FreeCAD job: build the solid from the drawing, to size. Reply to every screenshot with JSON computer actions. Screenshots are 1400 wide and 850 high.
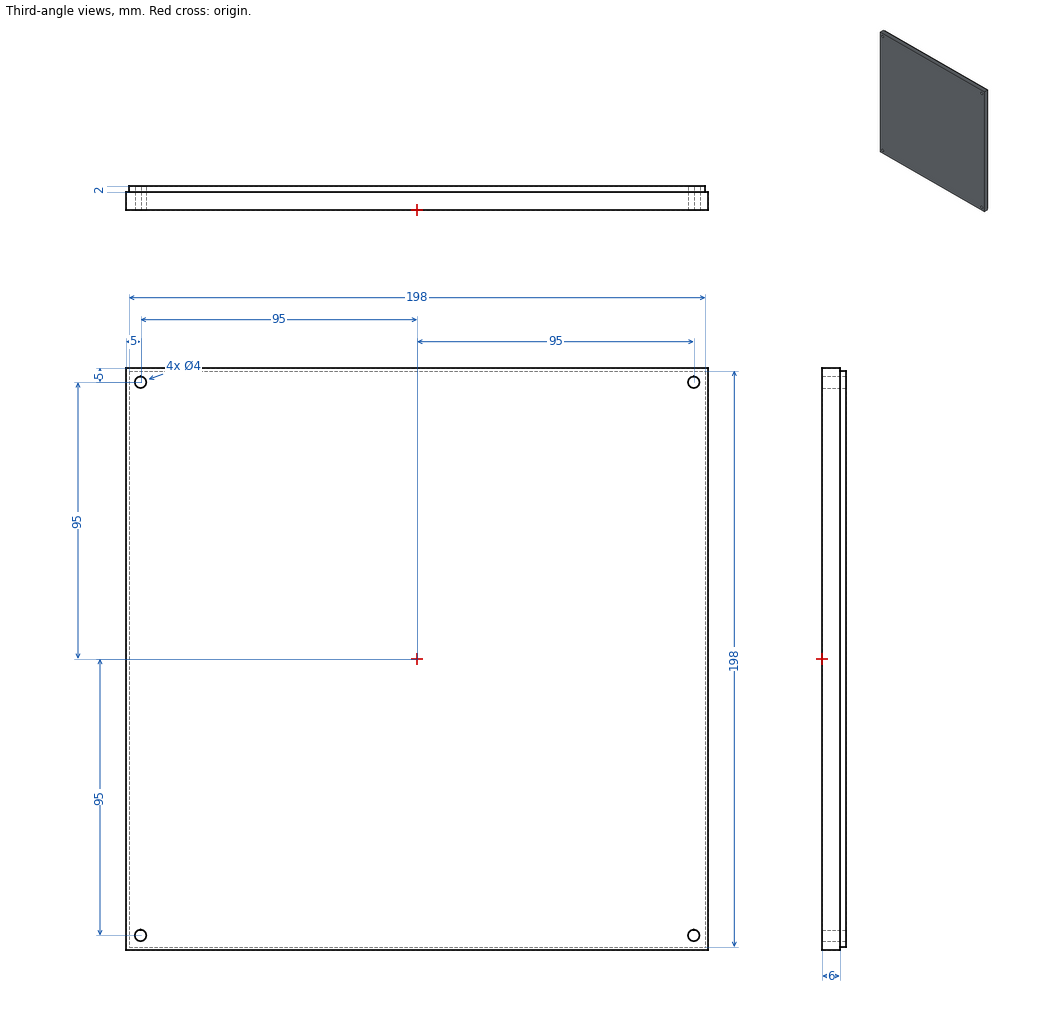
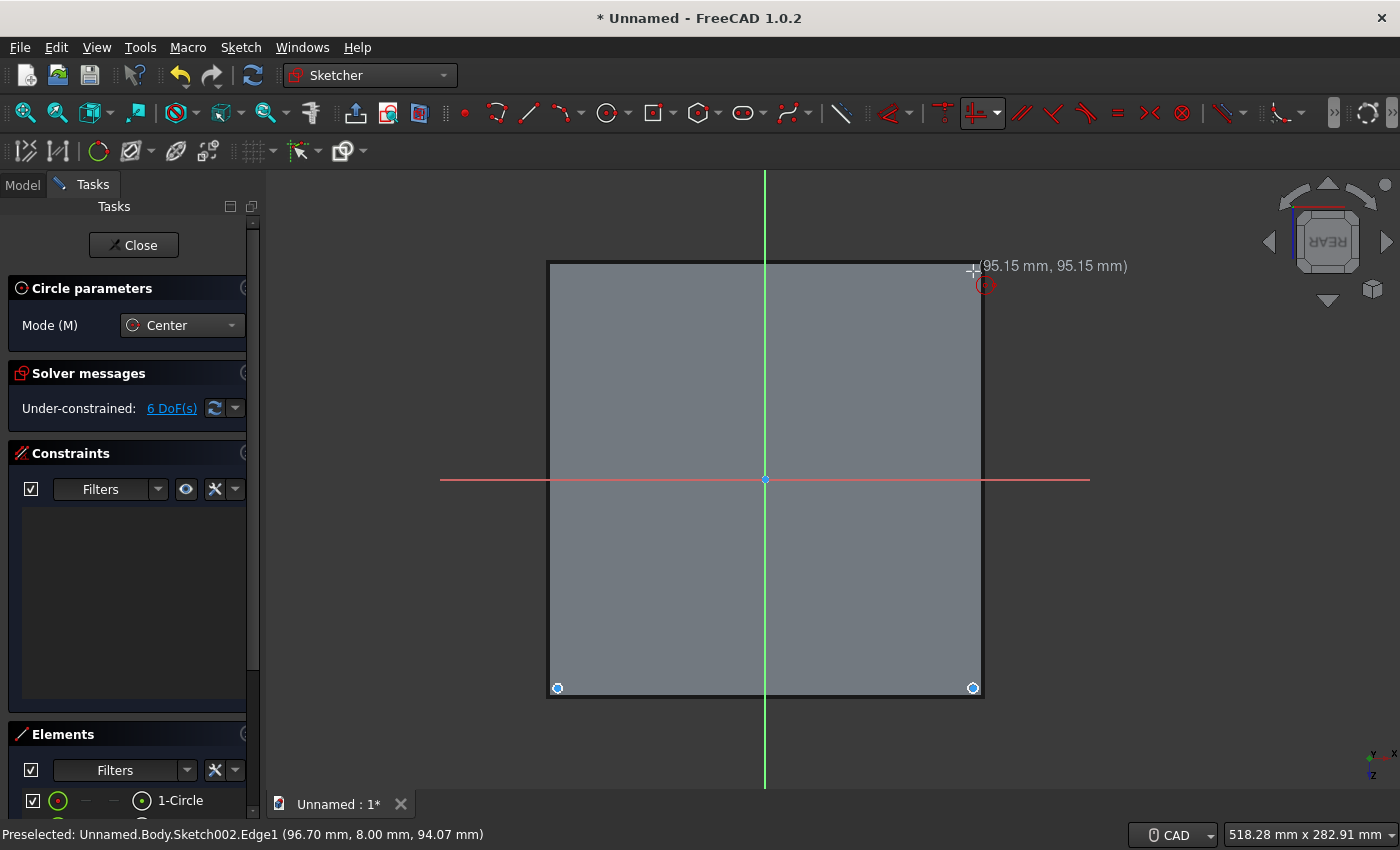
{"action": "left_click", "coordinate": [973, 272]}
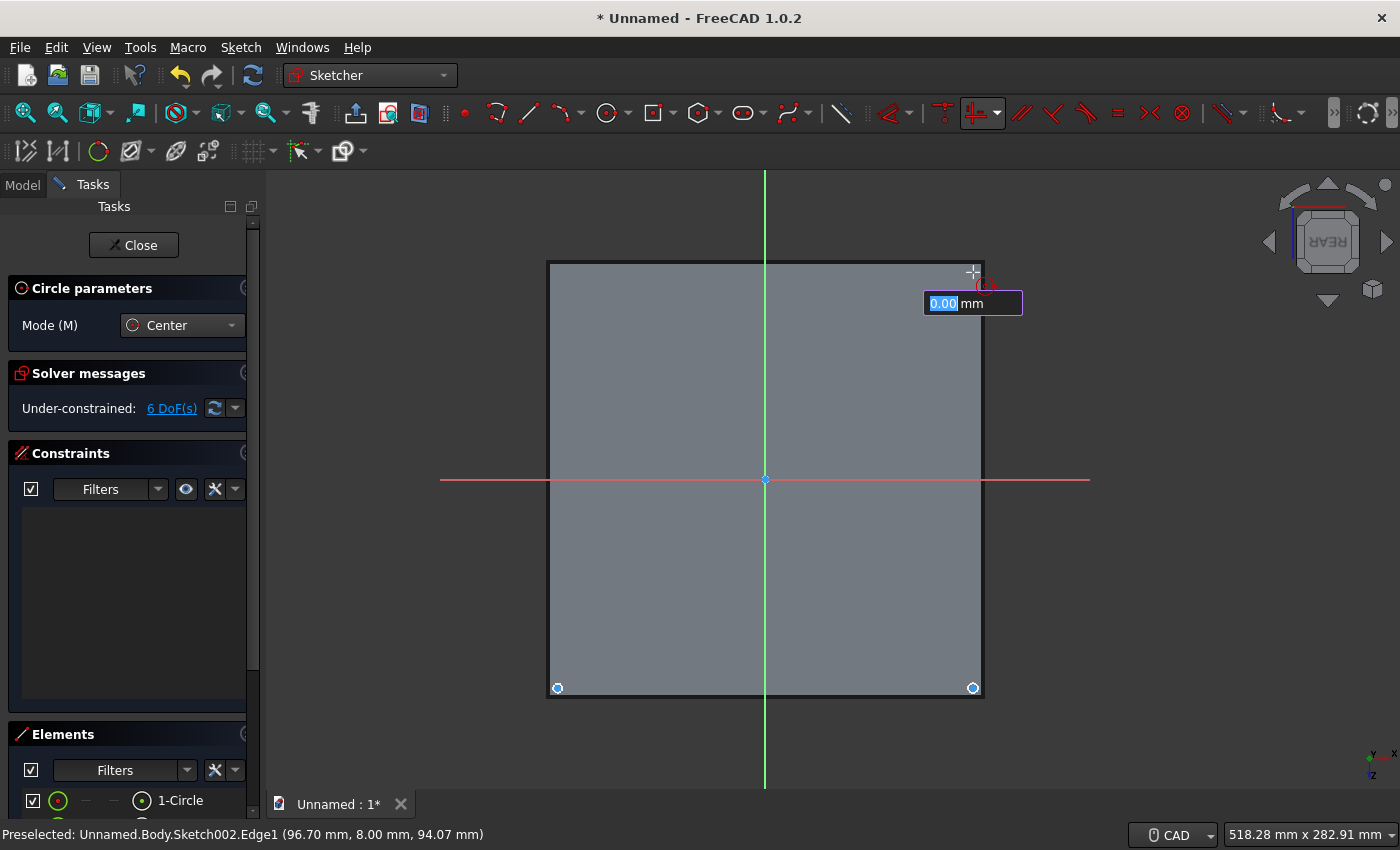
{"action": "scroll", "coordinate": [976, 269], "scroll_direction": "up", "scroll_amount": 7}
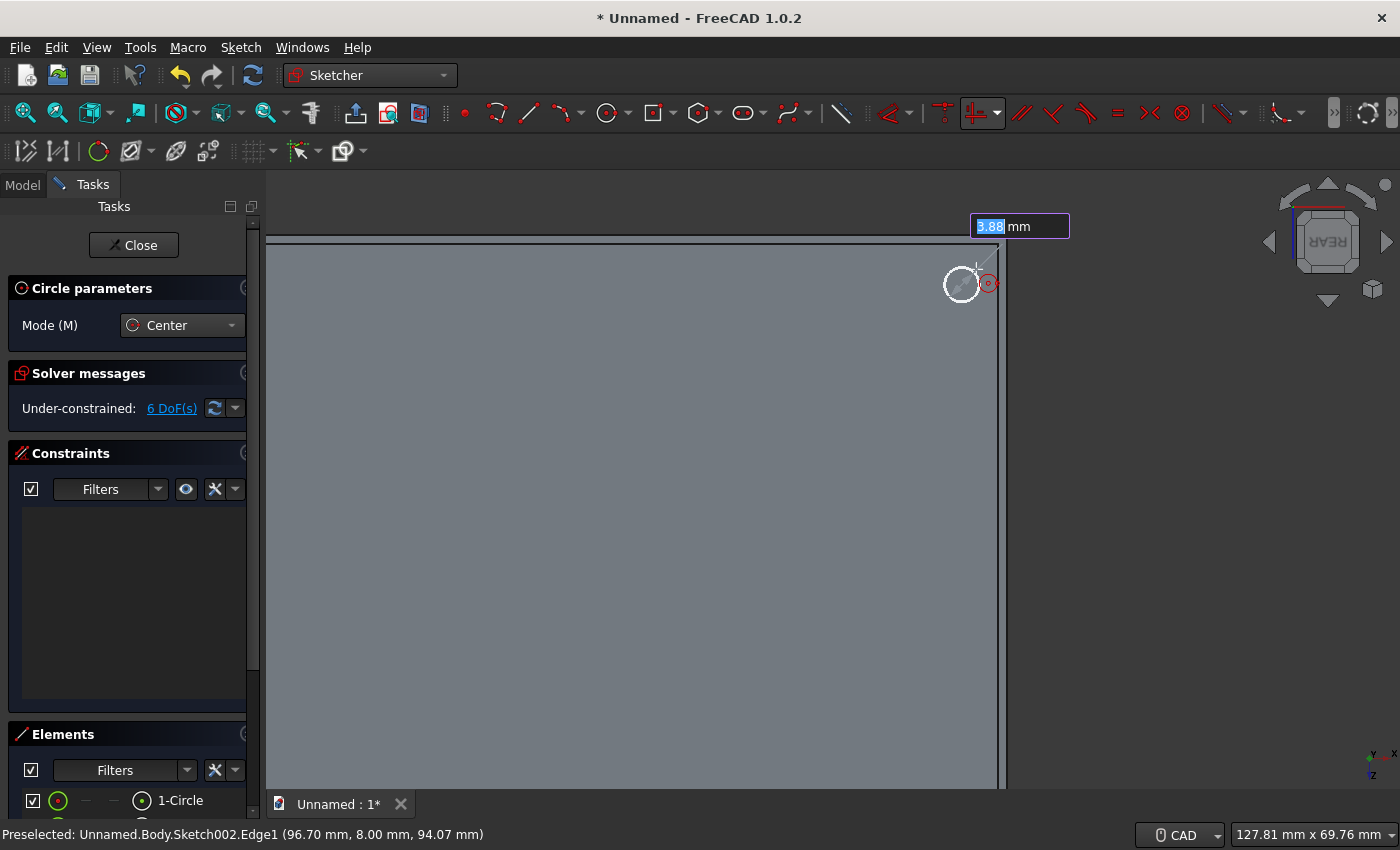
{"action": "left_click", "coordinate": [975, 267]}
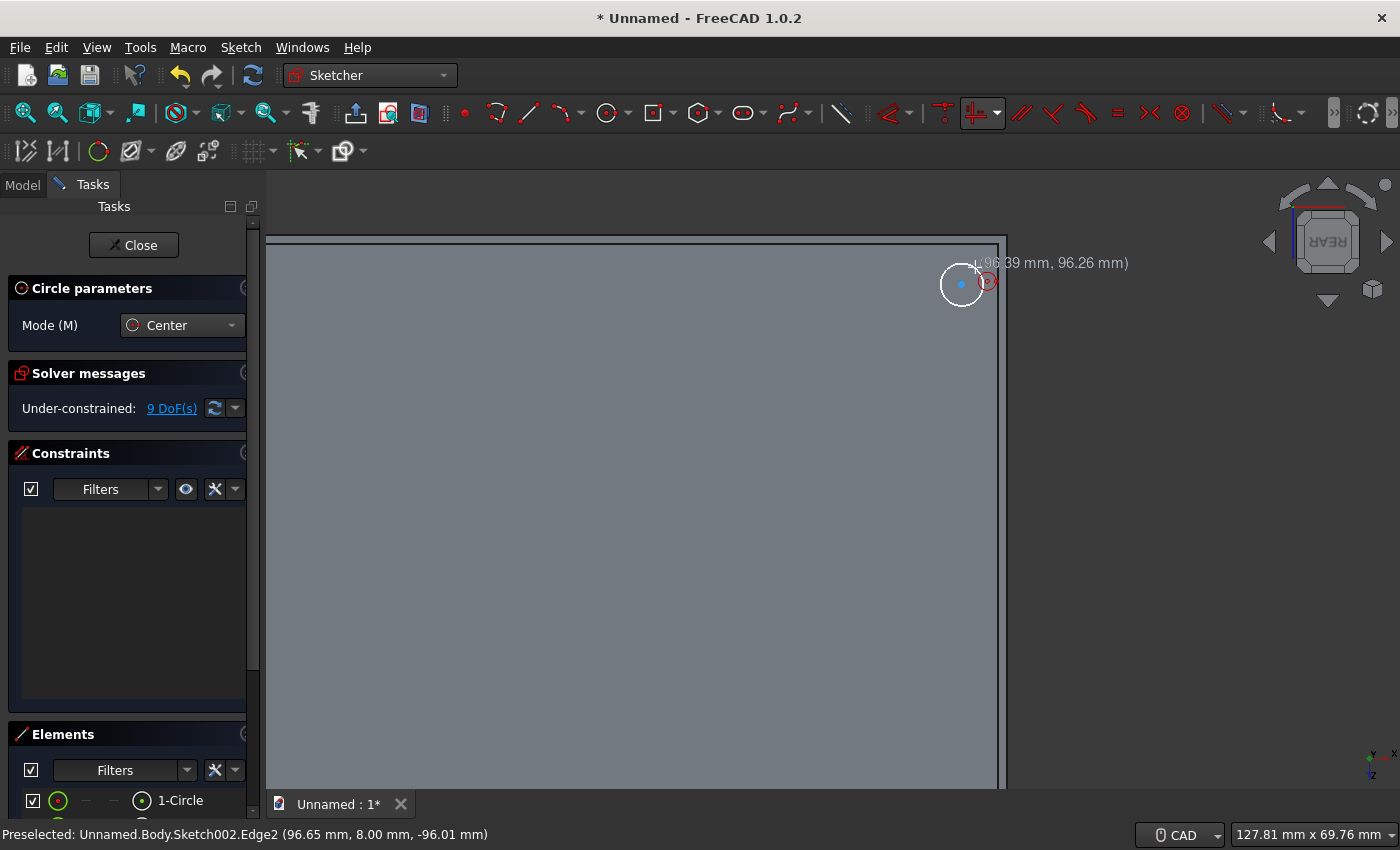
{"action": "scroll", "coordinate": [976, 269], "scroll_direction": "down", "scroll_amount": 7}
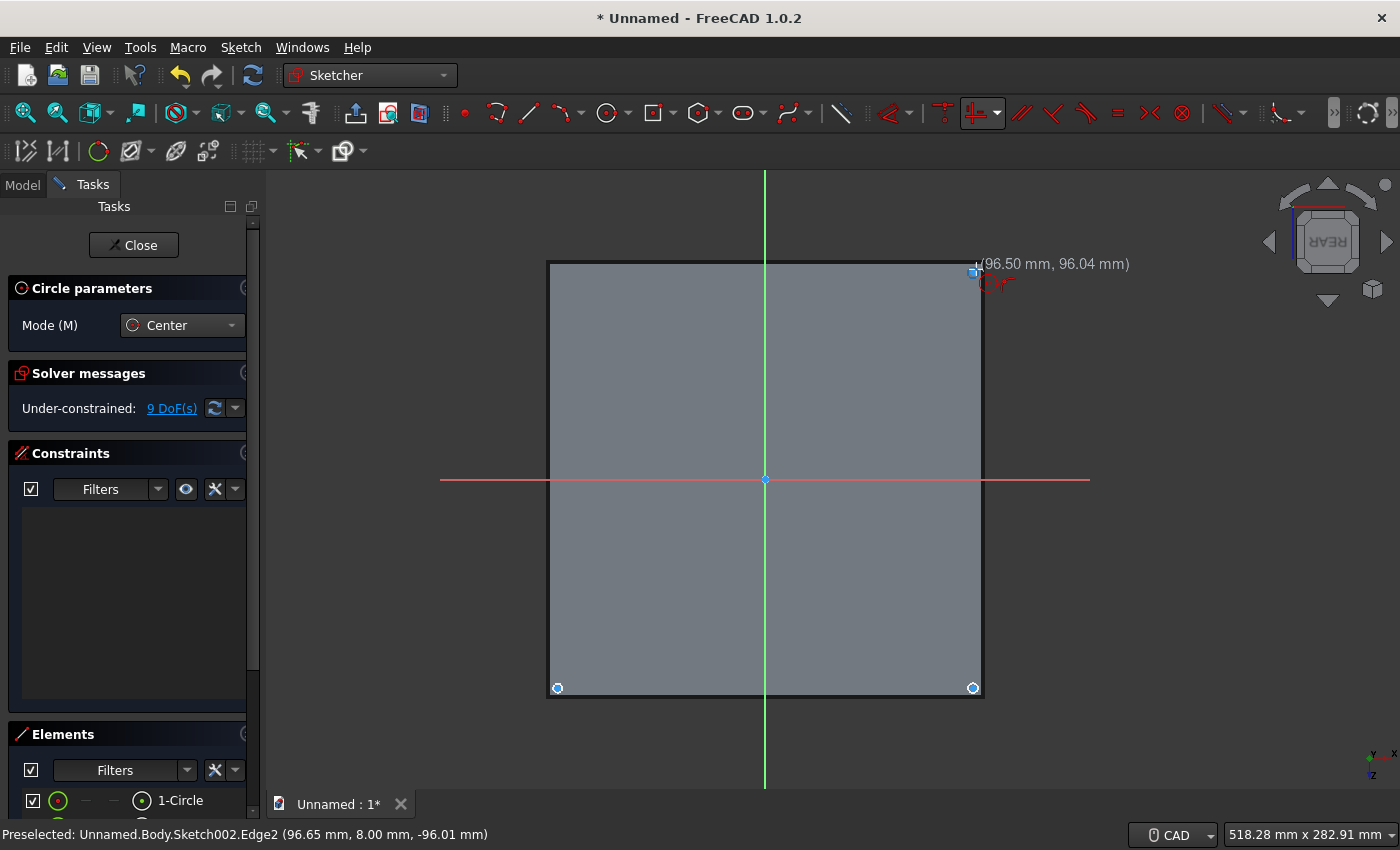
{"action": "scroll", "coordinate": [557, 272], "scroll_direction": "up", "scroll_amount": 9}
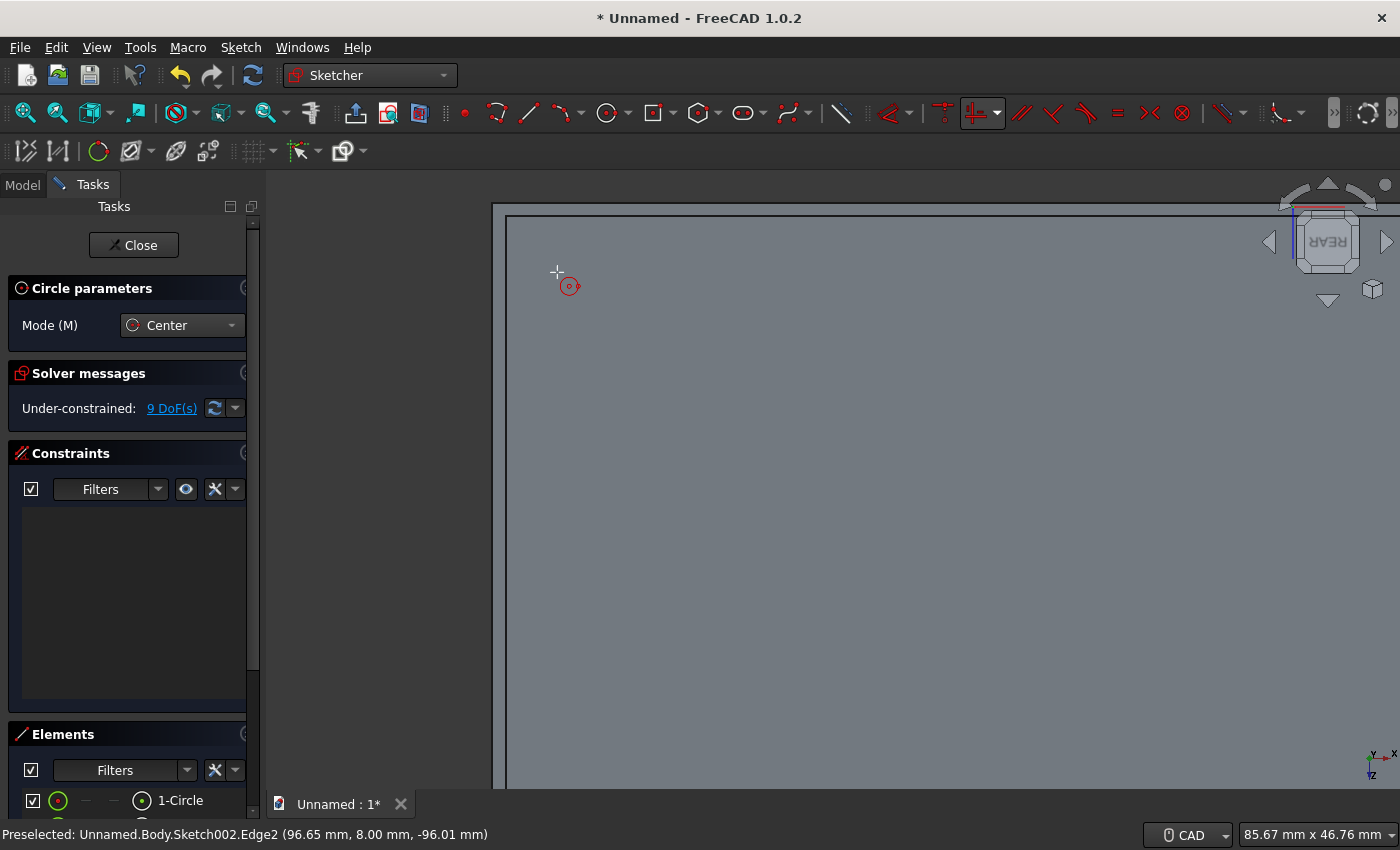
{"action": "scroll", "coordinate": [556, 272], "scroll_direction": "down", "scroll_amount": 9}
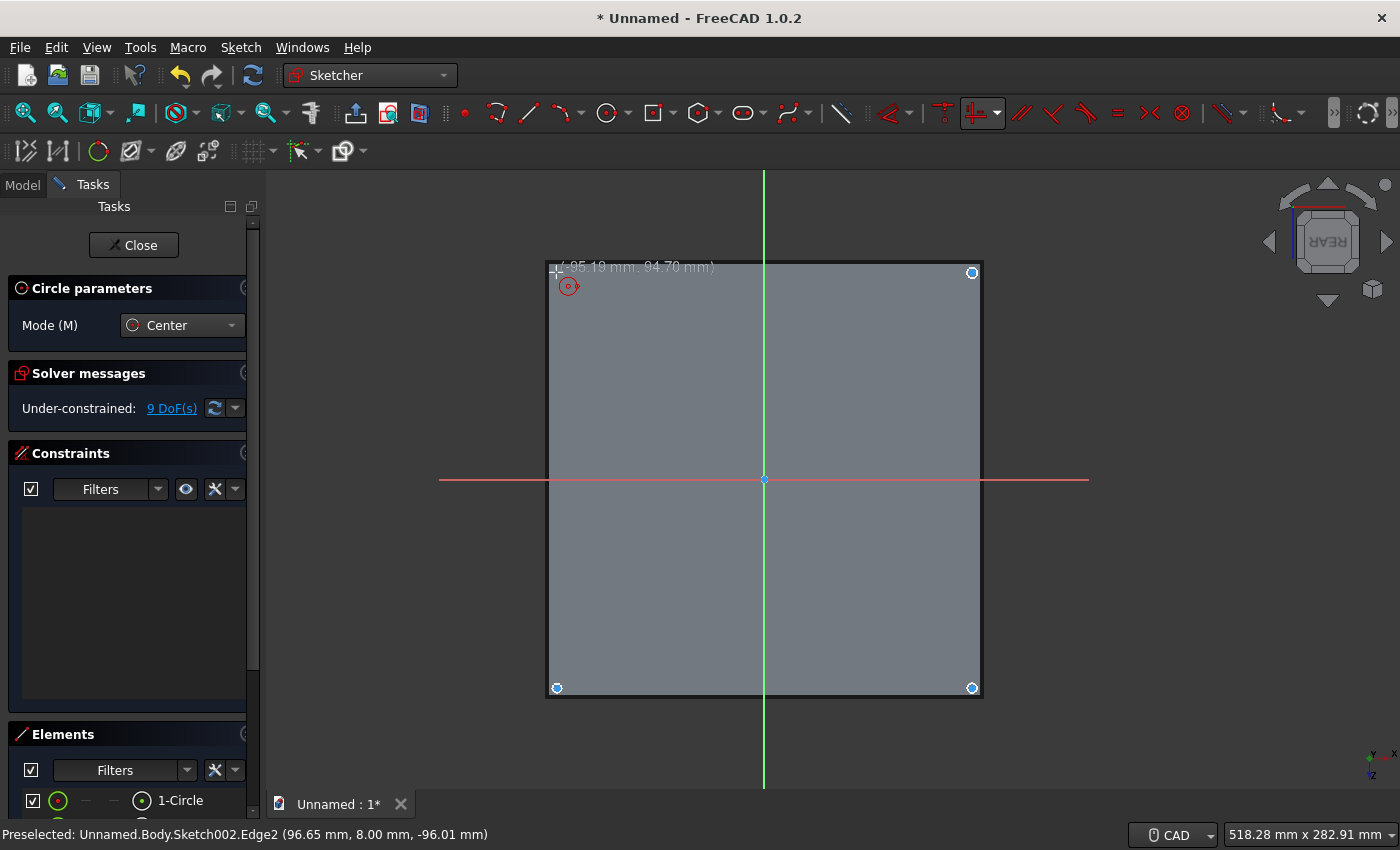
{"action": "left_click", "coordinate": [557, 272]}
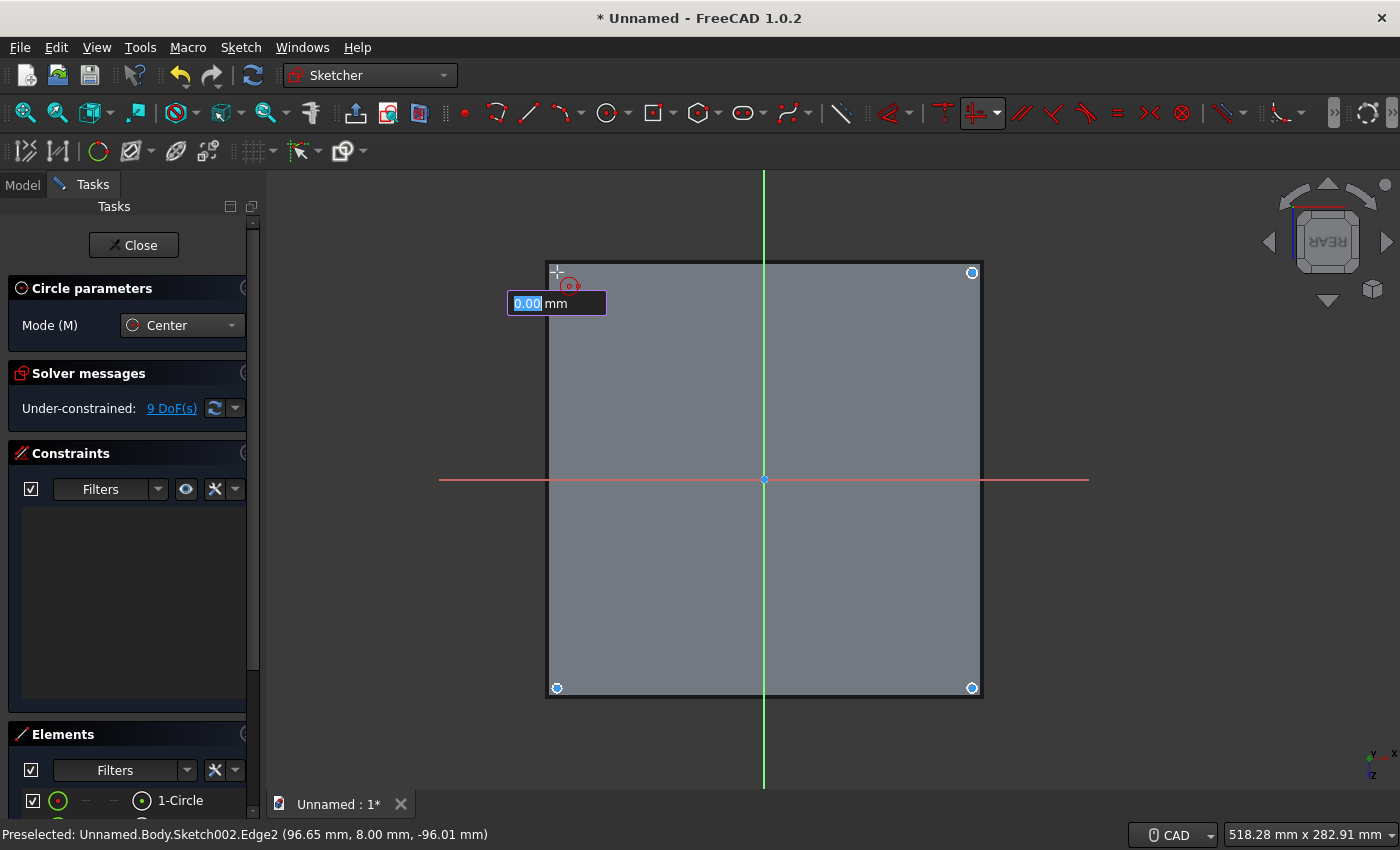
{"action": "scroll", "coordinate": [560, 269], "scroll_direction": "up", "scroll_amount": 7}